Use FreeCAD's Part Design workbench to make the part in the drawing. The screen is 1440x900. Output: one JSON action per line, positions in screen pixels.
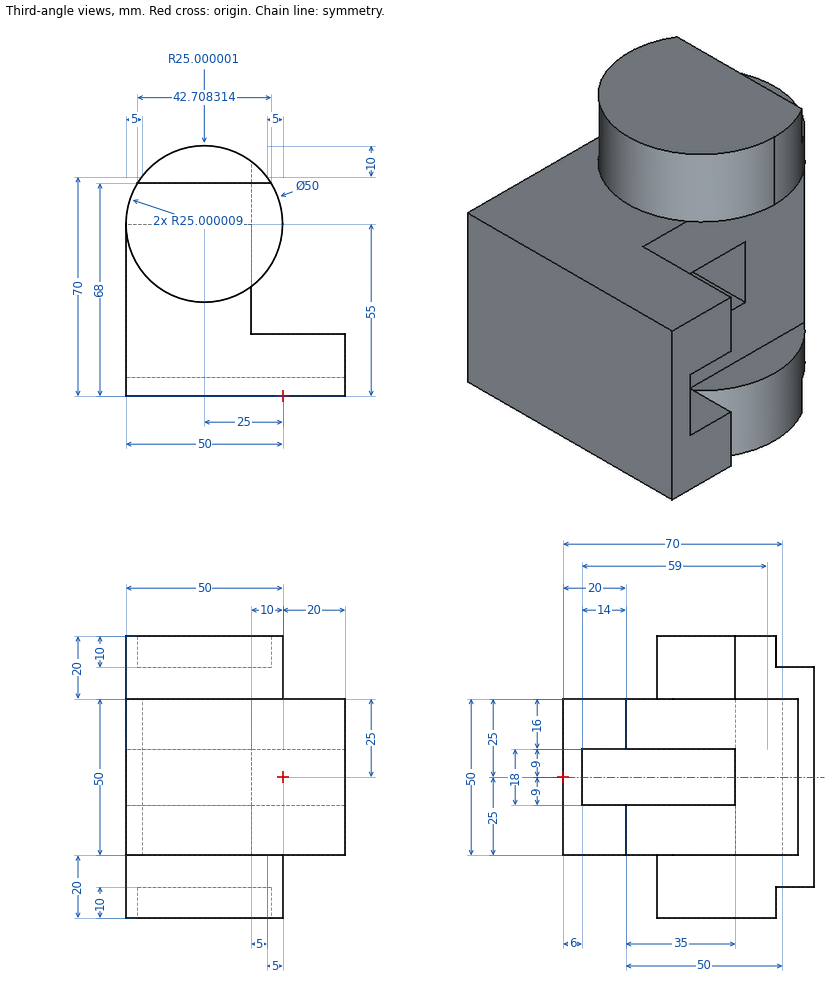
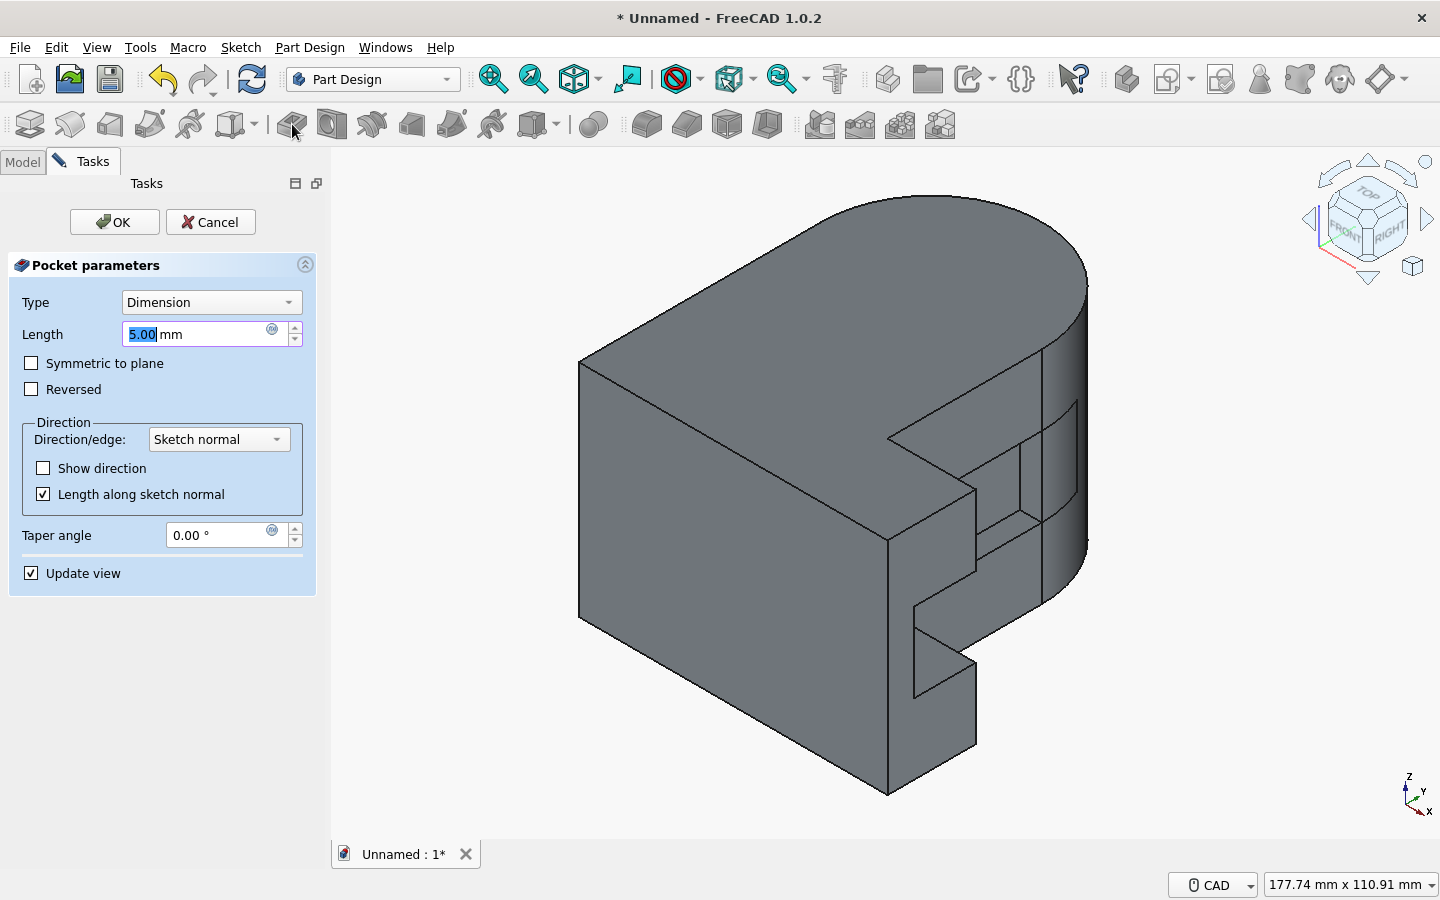
{"action": "type", "text": "50"}
{"action": "key", "text": "Tab"}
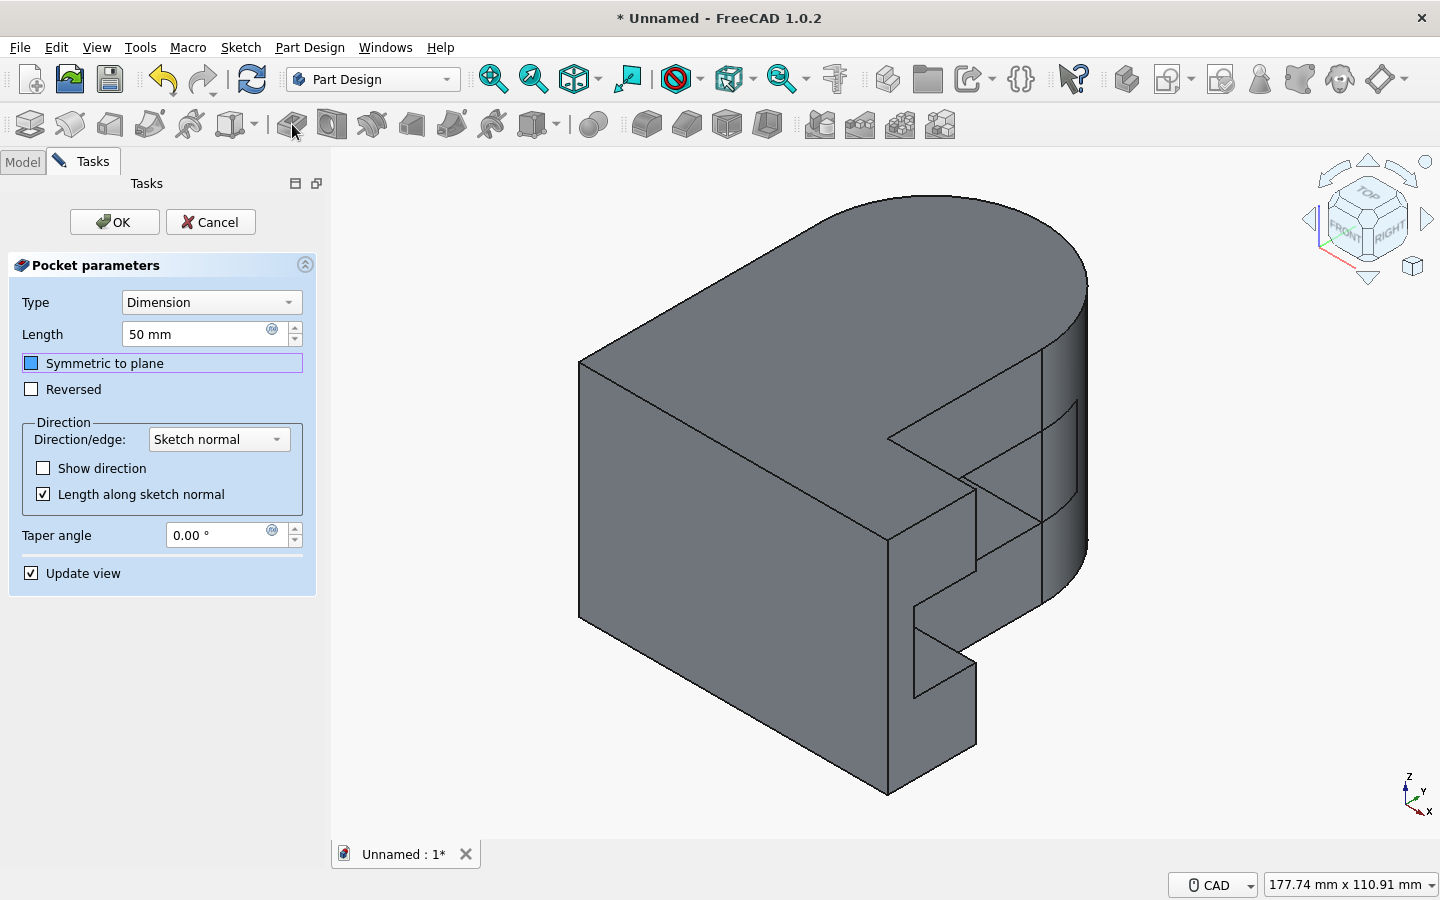
{"action": "left_click", "coordinate": [115, 222]}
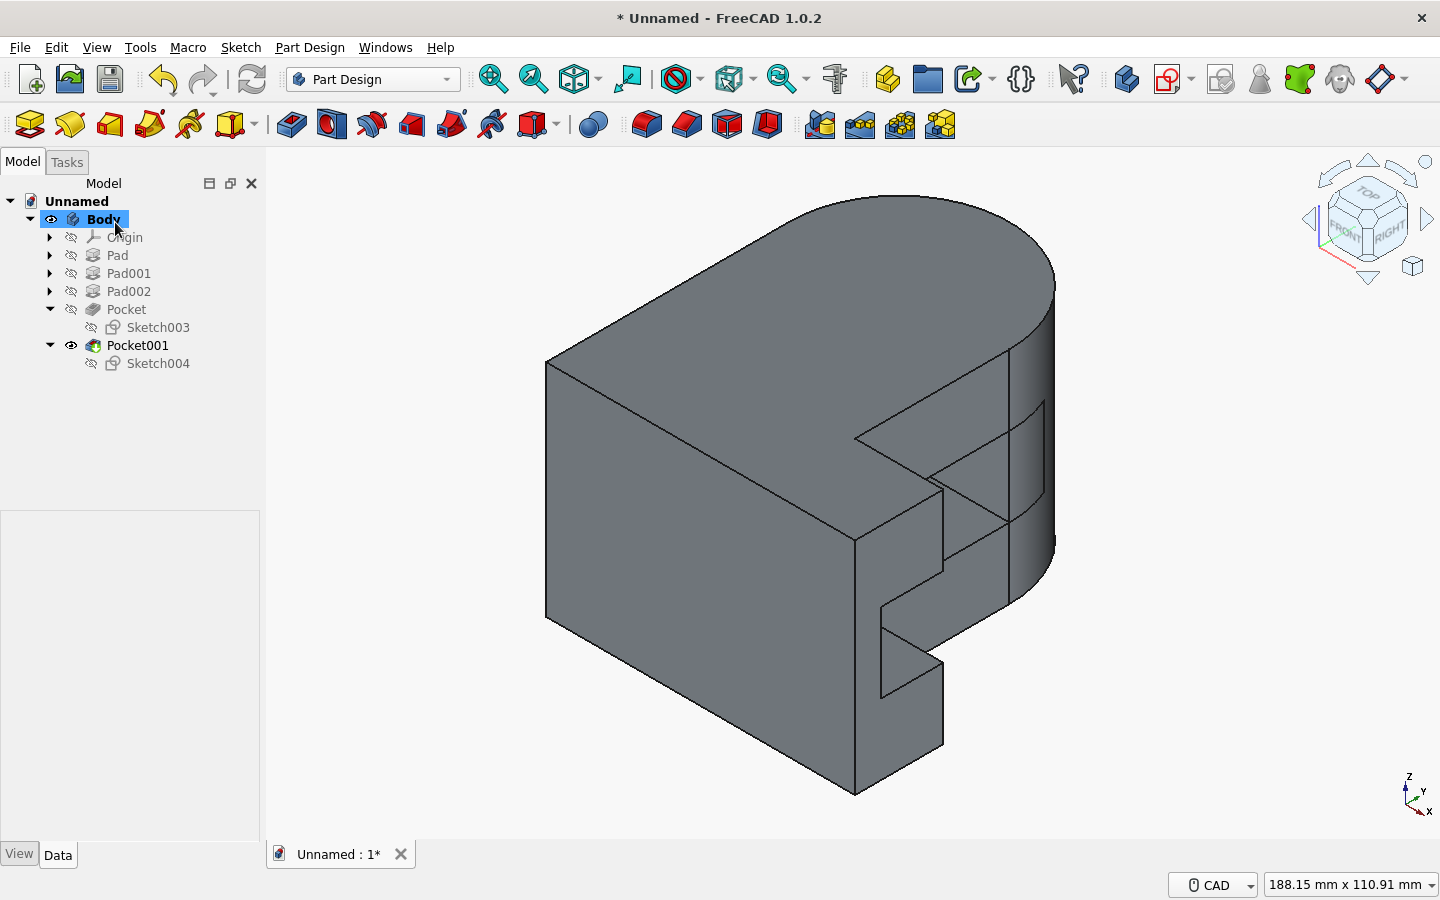
{"action": "left_click", "coordinate": [932, 607]}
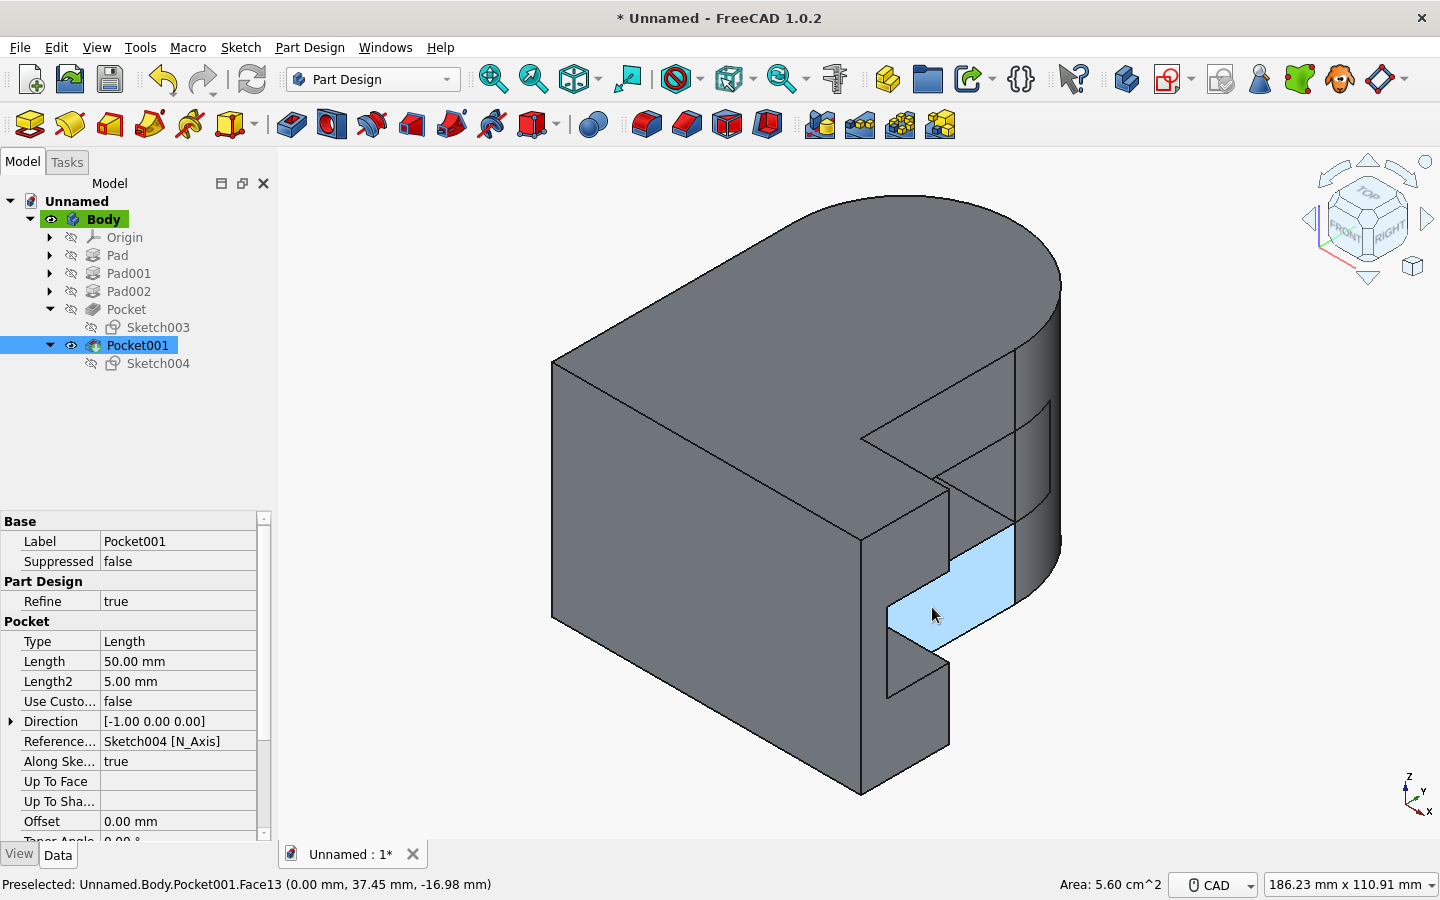
{"action": "left_click", "coordinate": [1168, 80]}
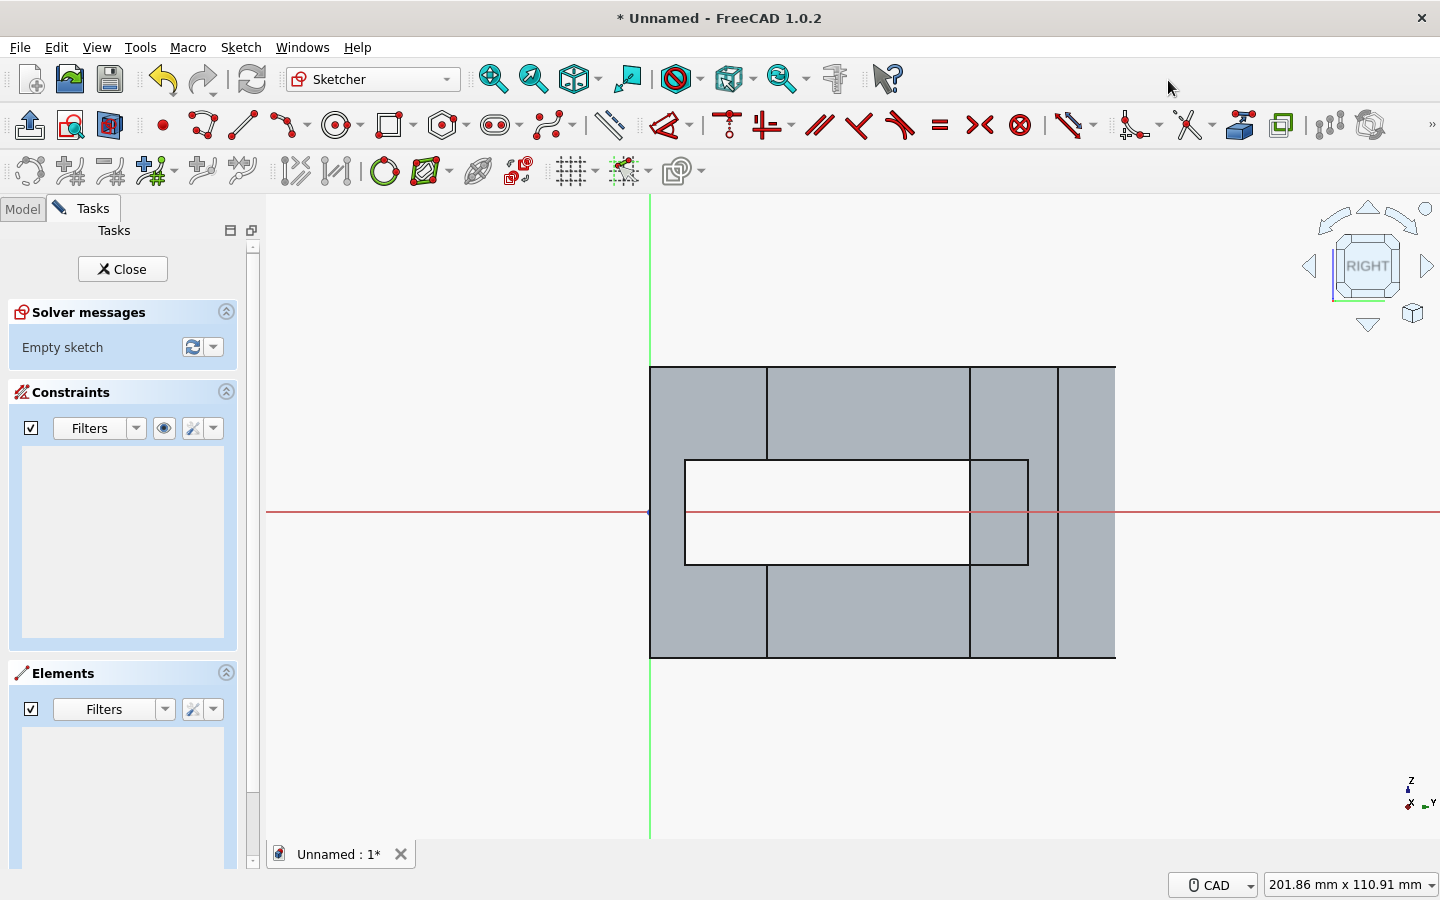
{"action": "left_click", "coordinate": [110, 126]}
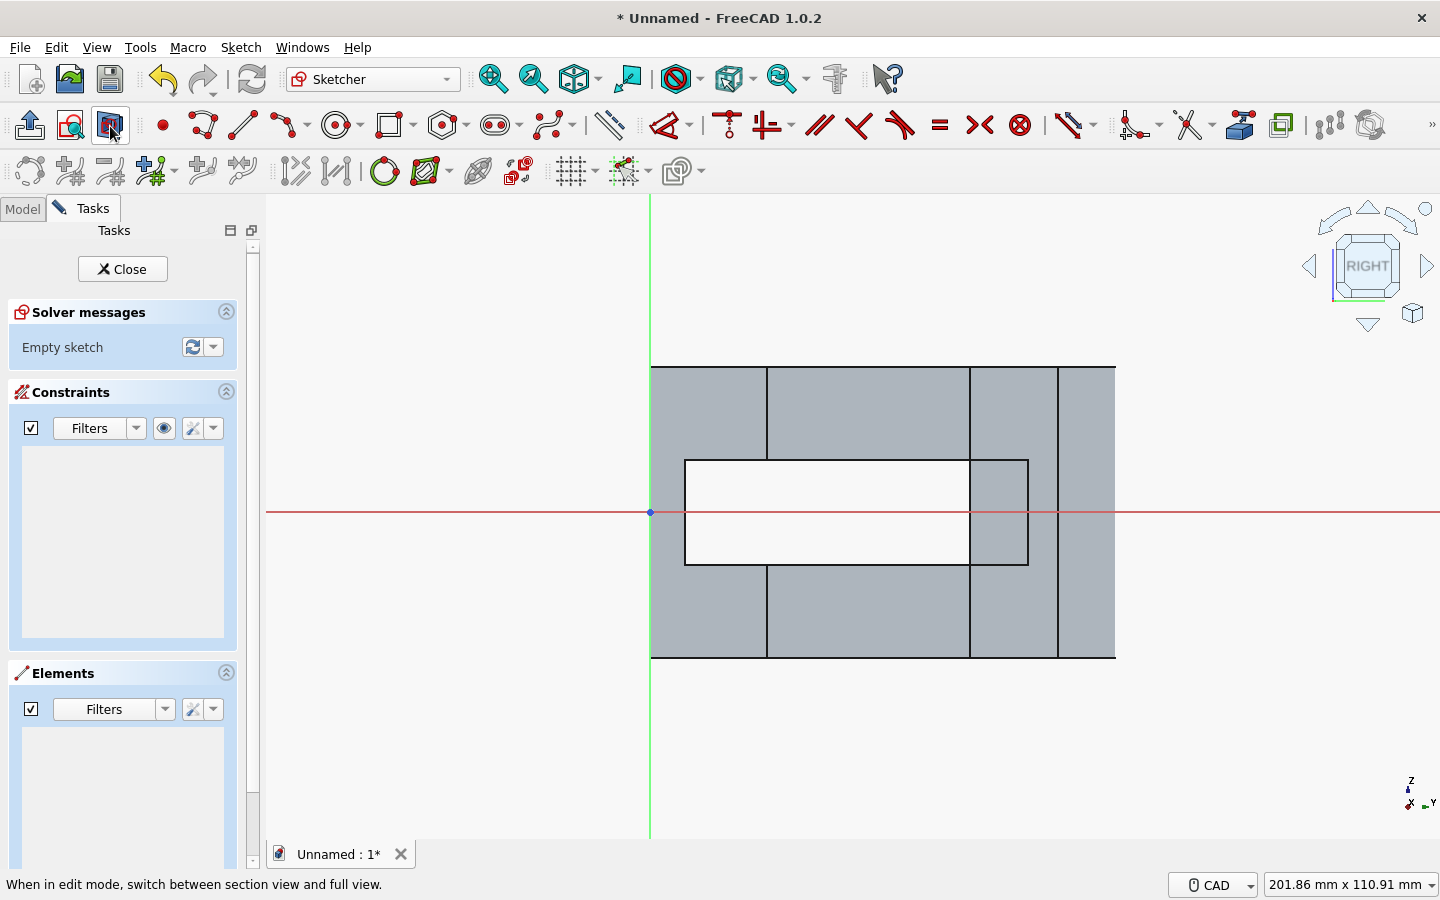
{"action": "scroll", "coordinate": [995, 503], "scroll_direction": "up", "scroll_amount": 2}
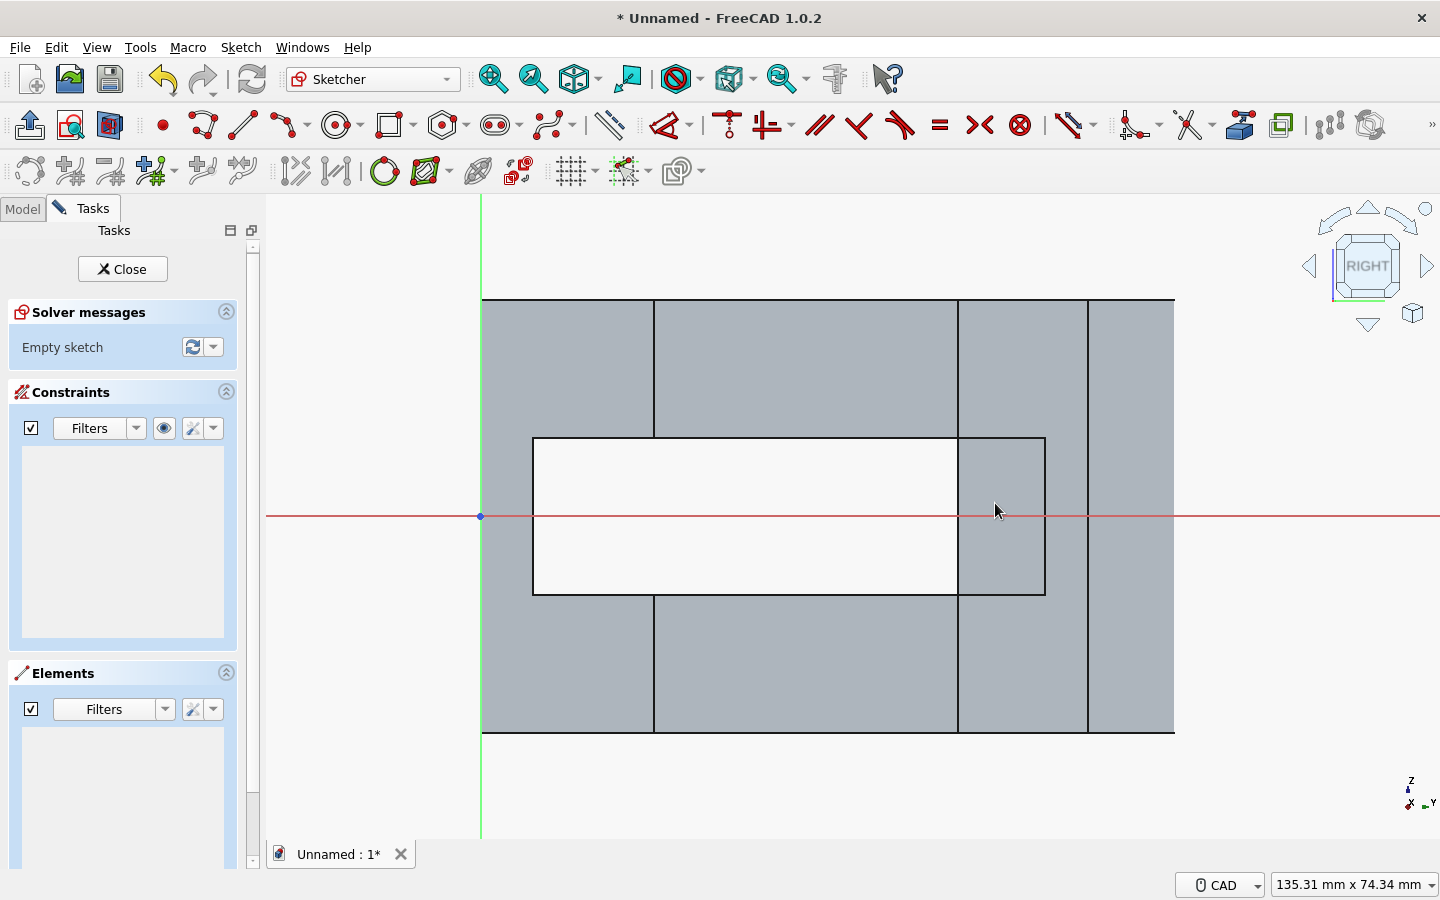
{"action": "left_click", "coordinate": [390, 126]}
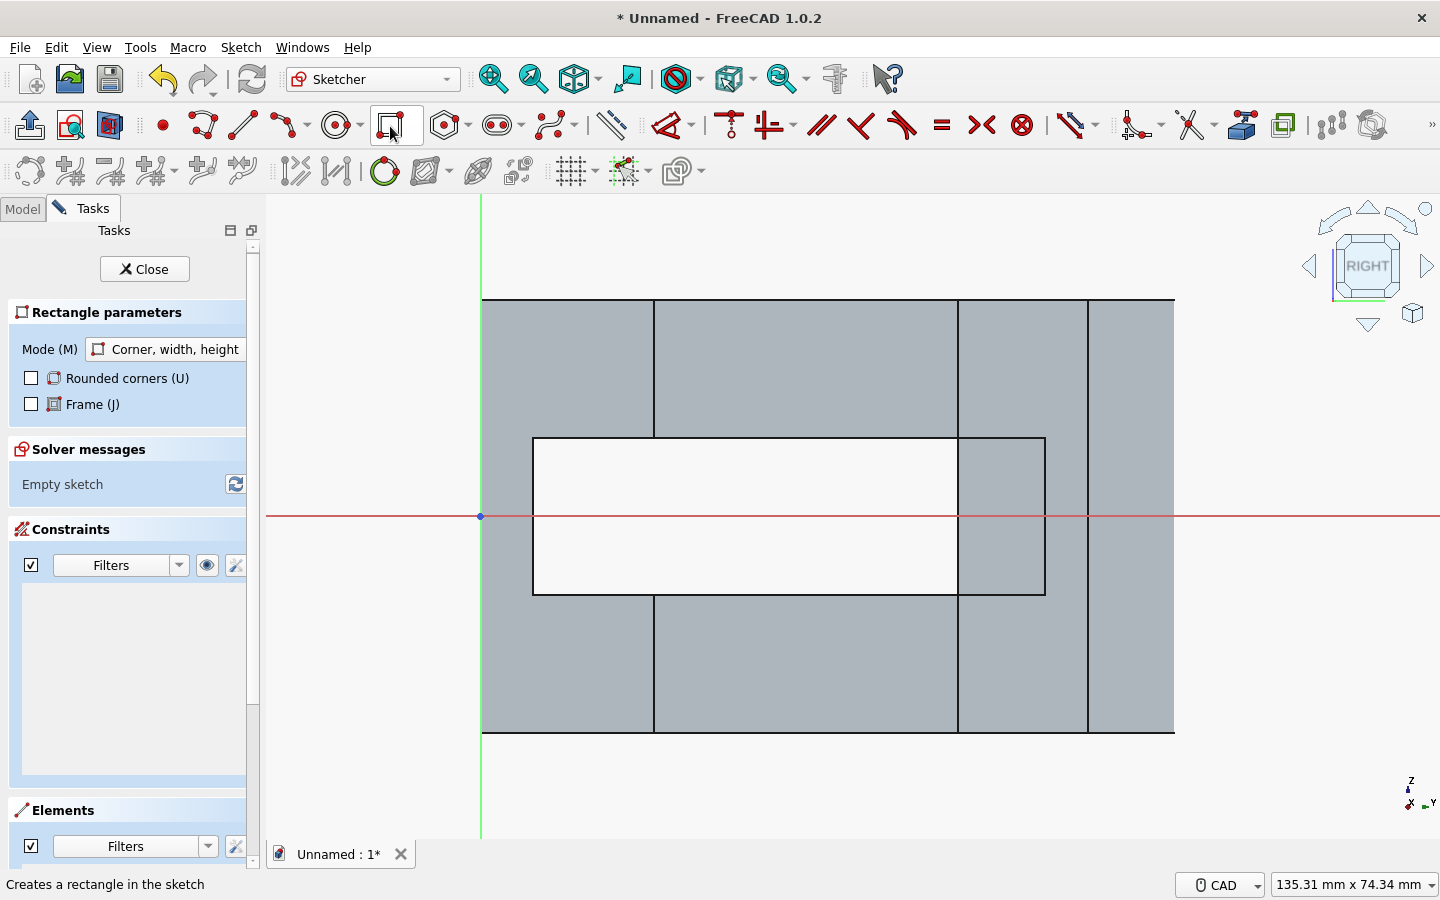
{"action": "left_click", "coordinate": [654, 300]}
{"action": "mouse_move", "coordinate": [1088, 733]}